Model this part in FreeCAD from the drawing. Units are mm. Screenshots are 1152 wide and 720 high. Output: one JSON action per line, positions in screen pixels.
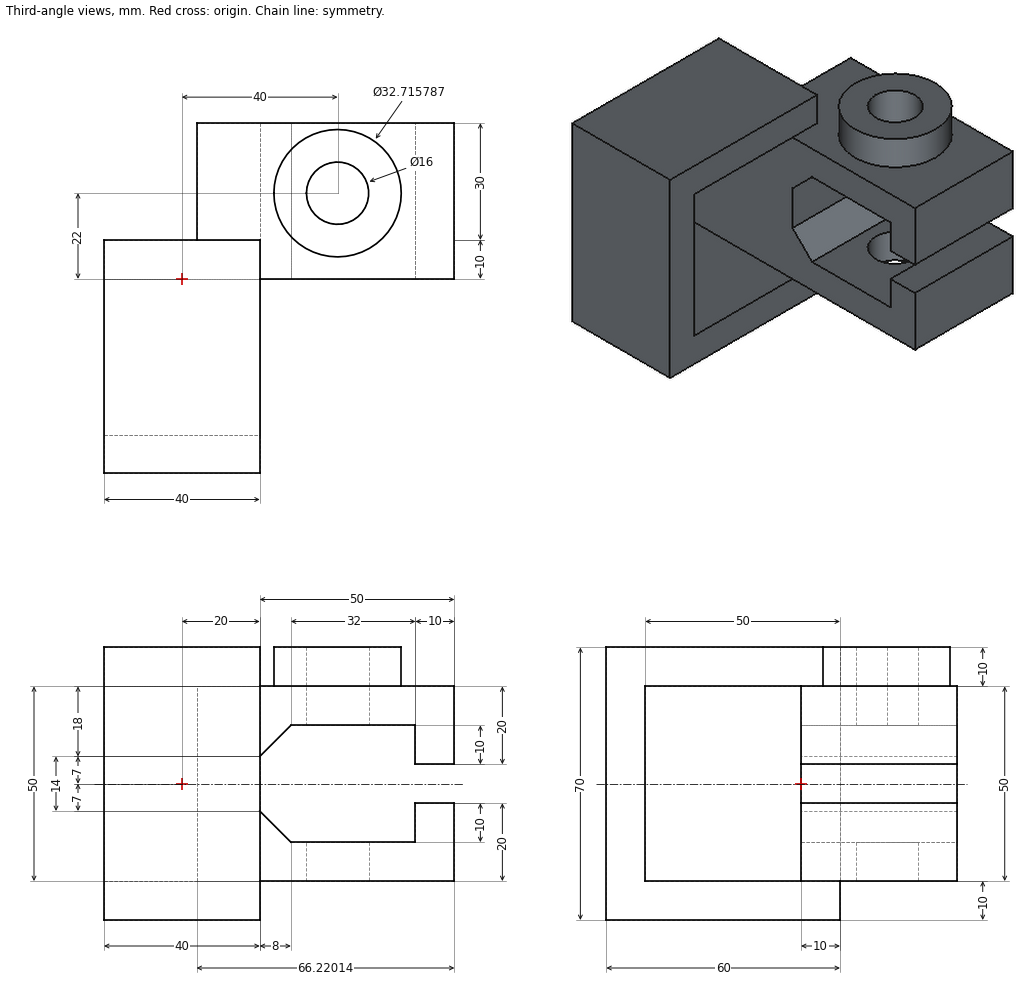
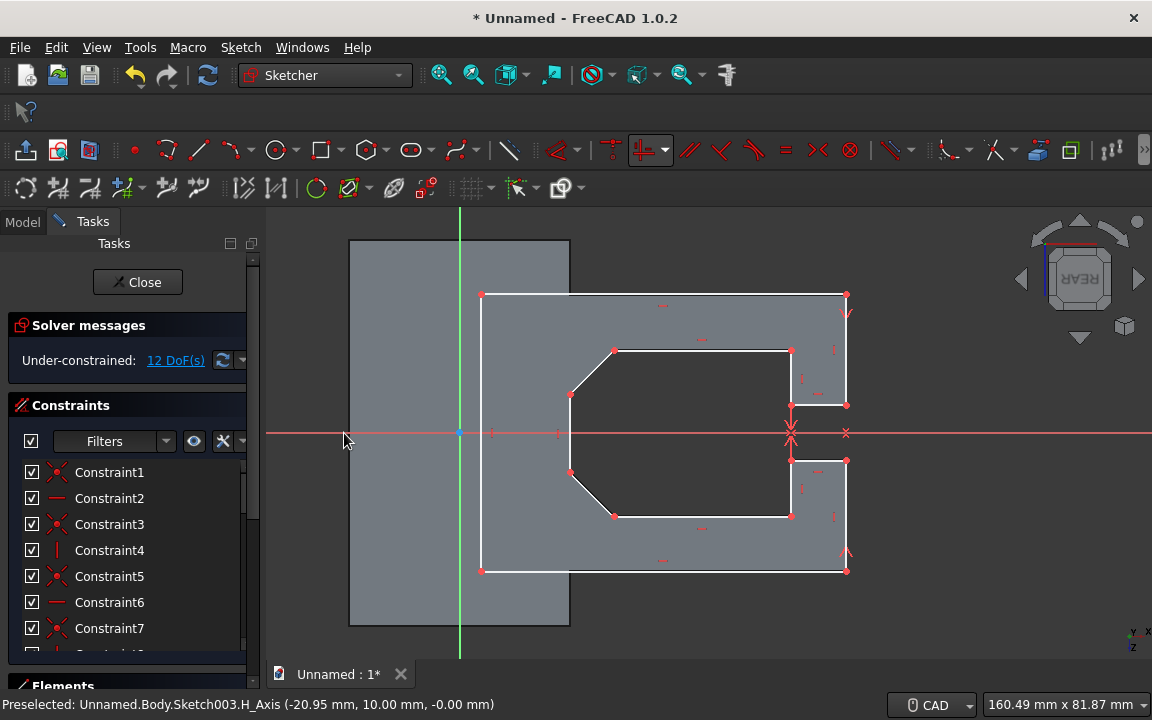
{"action": "left_click", "coordinate": [614, 351]}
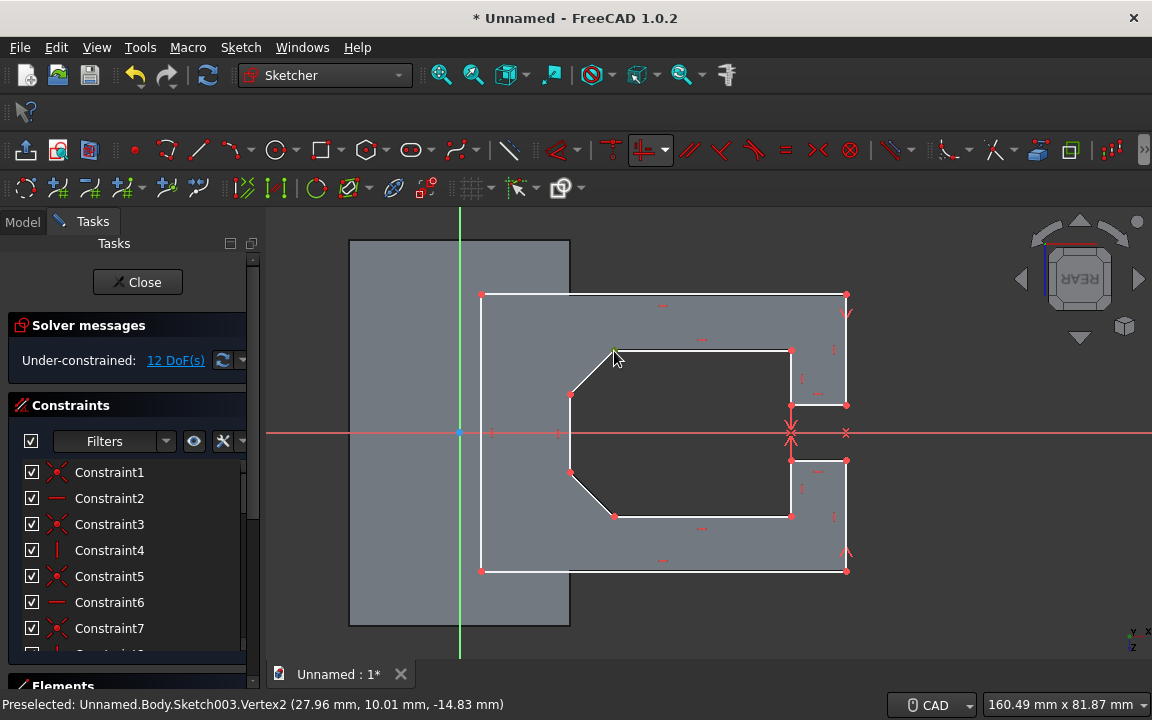
{"action": "left_click", "coordinate": [614, 517]}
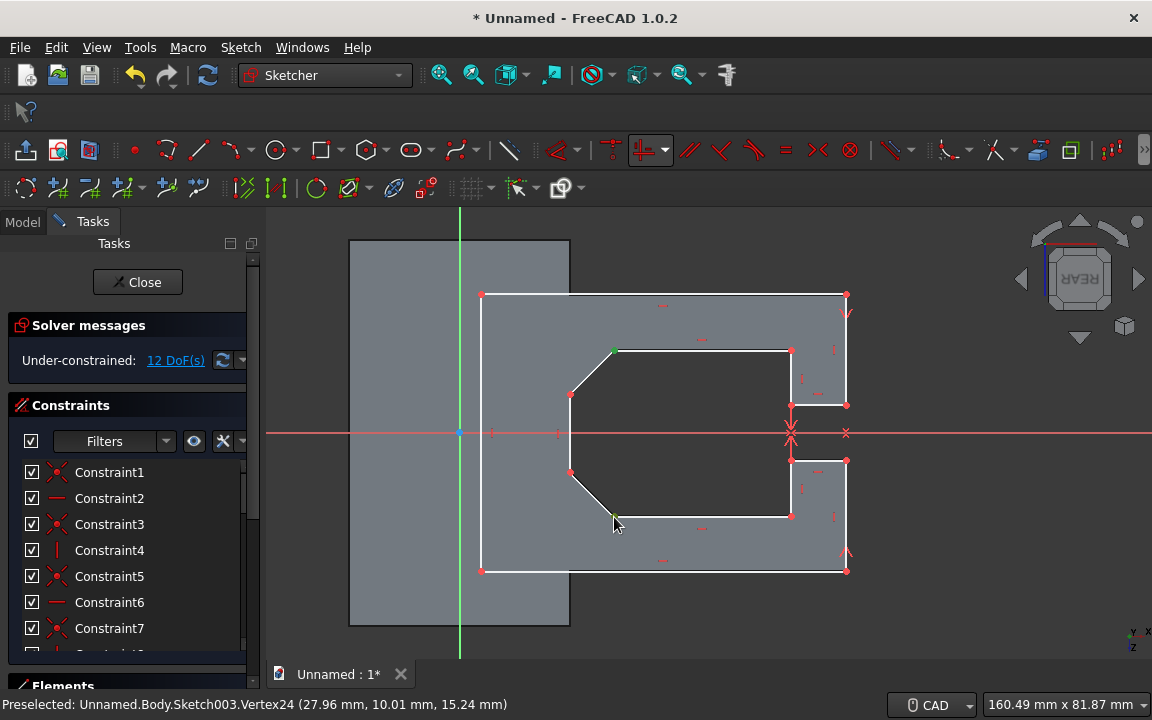
{"action": "left_click", "coordinate": [344, 433]}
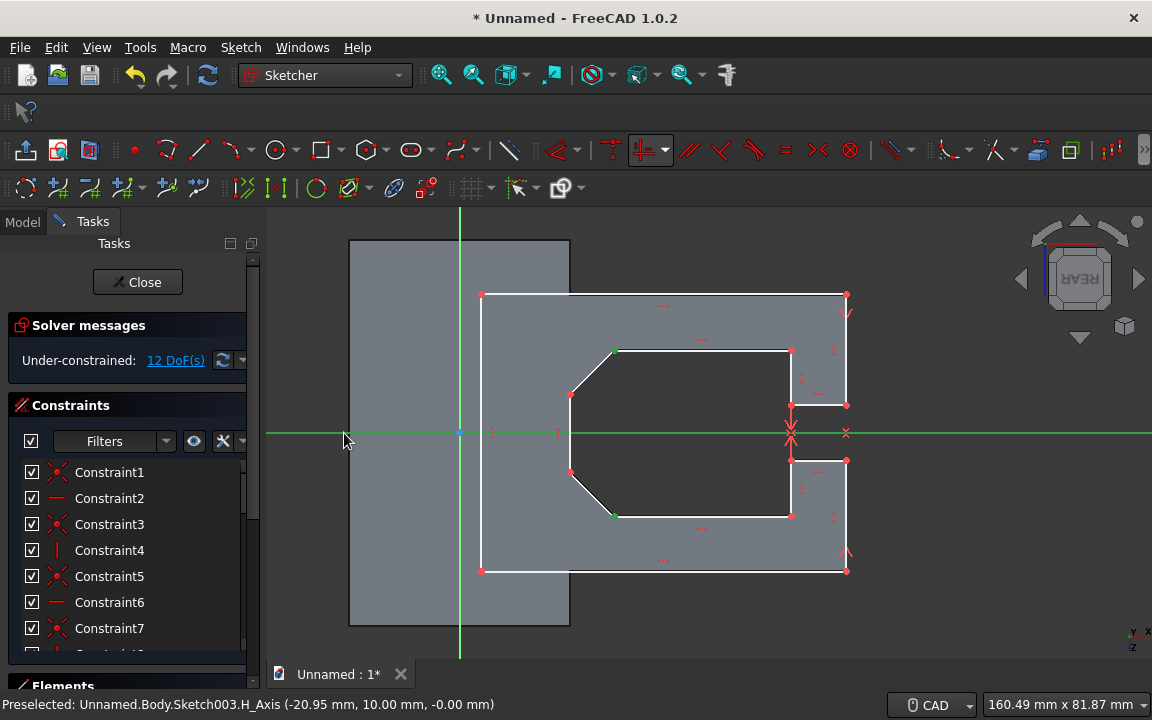
{"action": "key", "text": "s"}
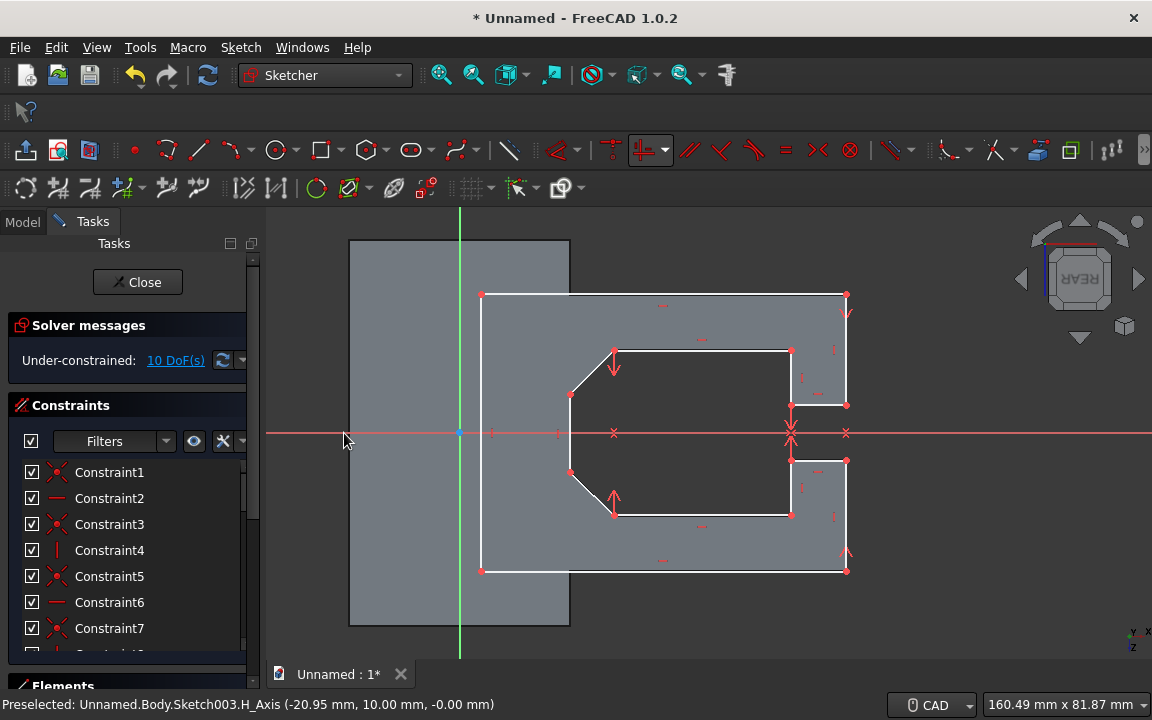
{"action": "key", "text": "d"}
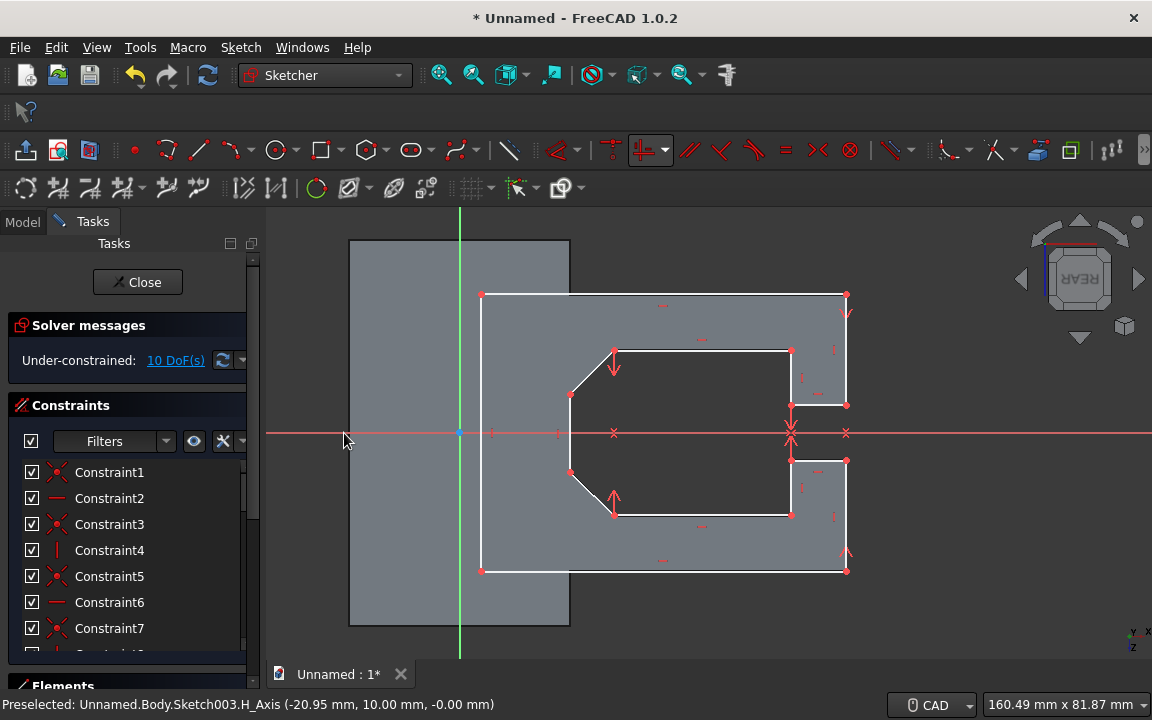
{"action": "left_click", "coordinate": [667, 351]}
{"action": "left_click", "coordinate": [703, 317]}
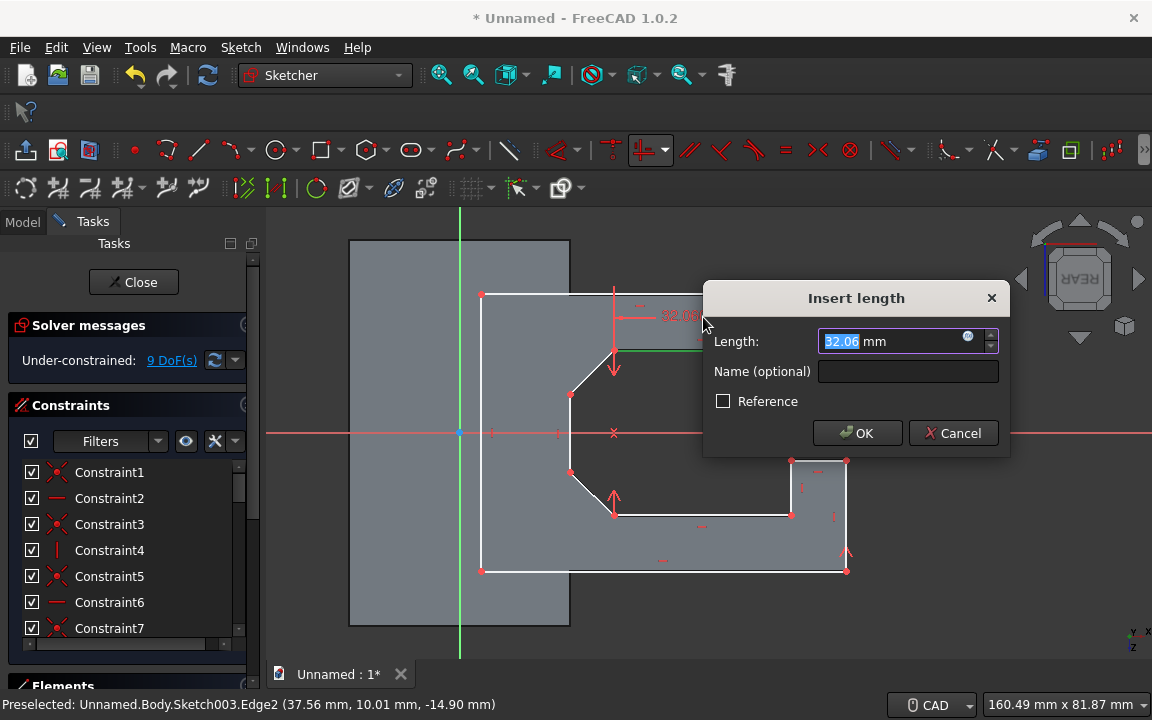
{"action": "type", "text": "32"}
{"action": "key", "text": "Return"}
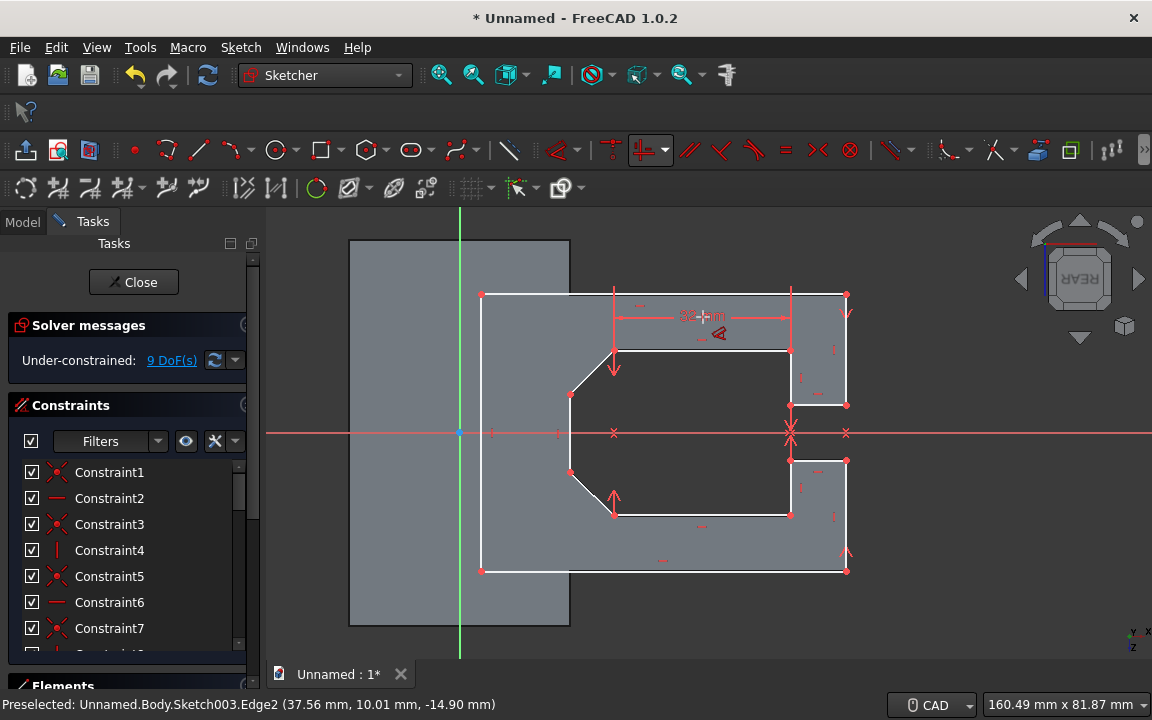
{"action": "left_click", "coordinate": [791, 367]}
{"action": "left_click", "coordinate": [825, 378]}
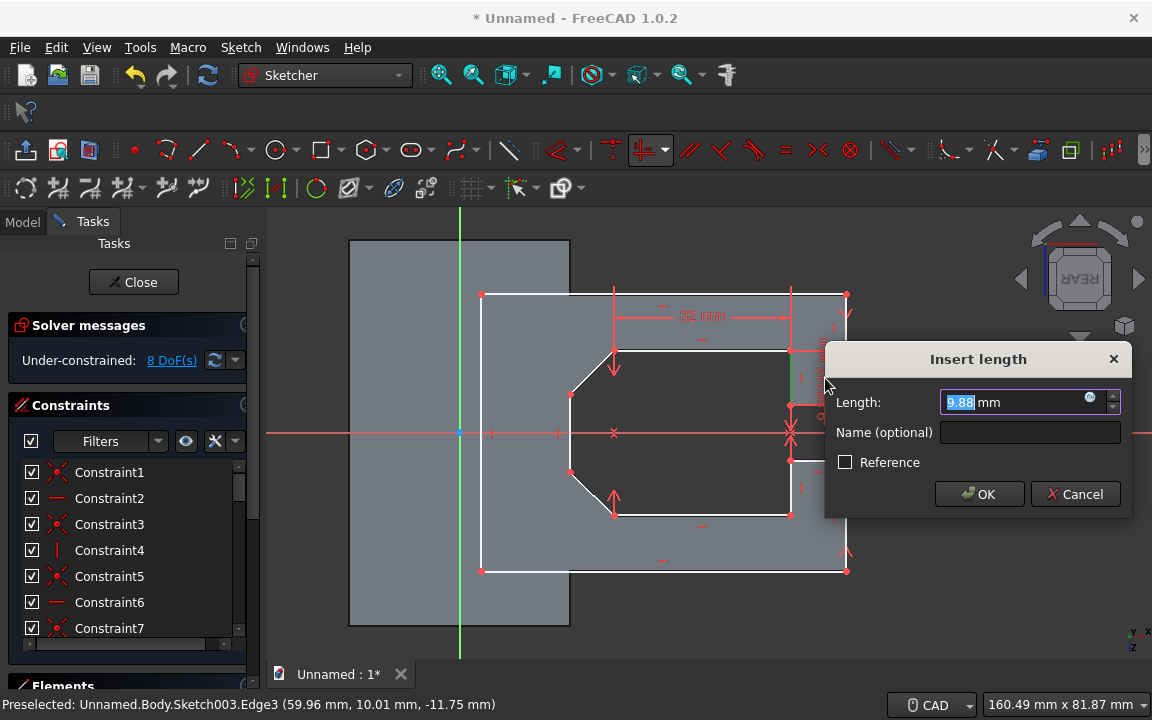
{"action": "type", "text": "10"}
{"action": "key", "text": "Return"}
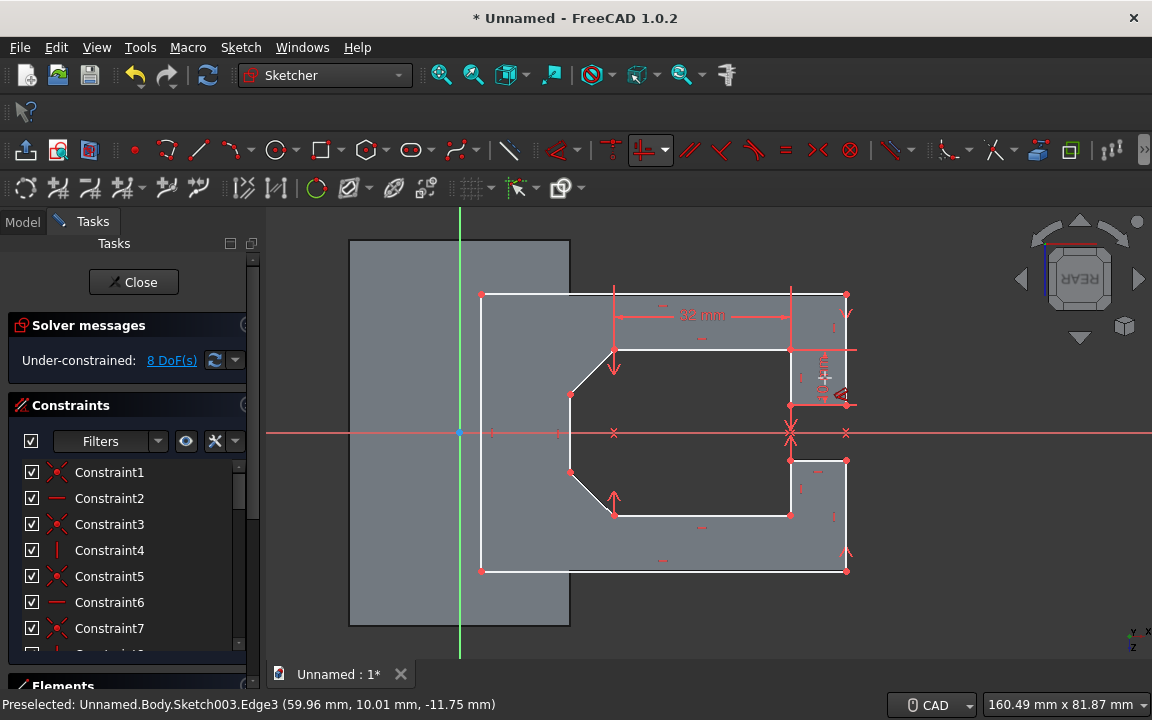
{"action": "left_click", "coordinate": [807, 405]}
{"action": "left_click", "coordinate": [818, 347]}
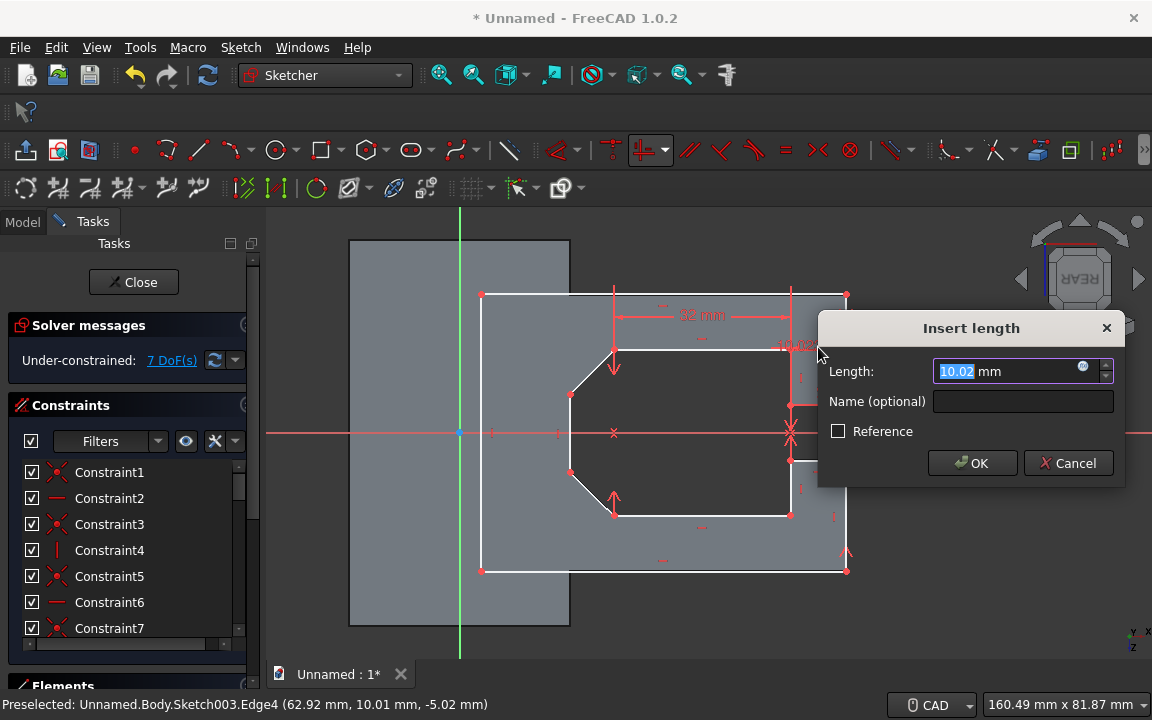
{"action": "type", "text": "10"}
{"action": "key", "text": "Return"}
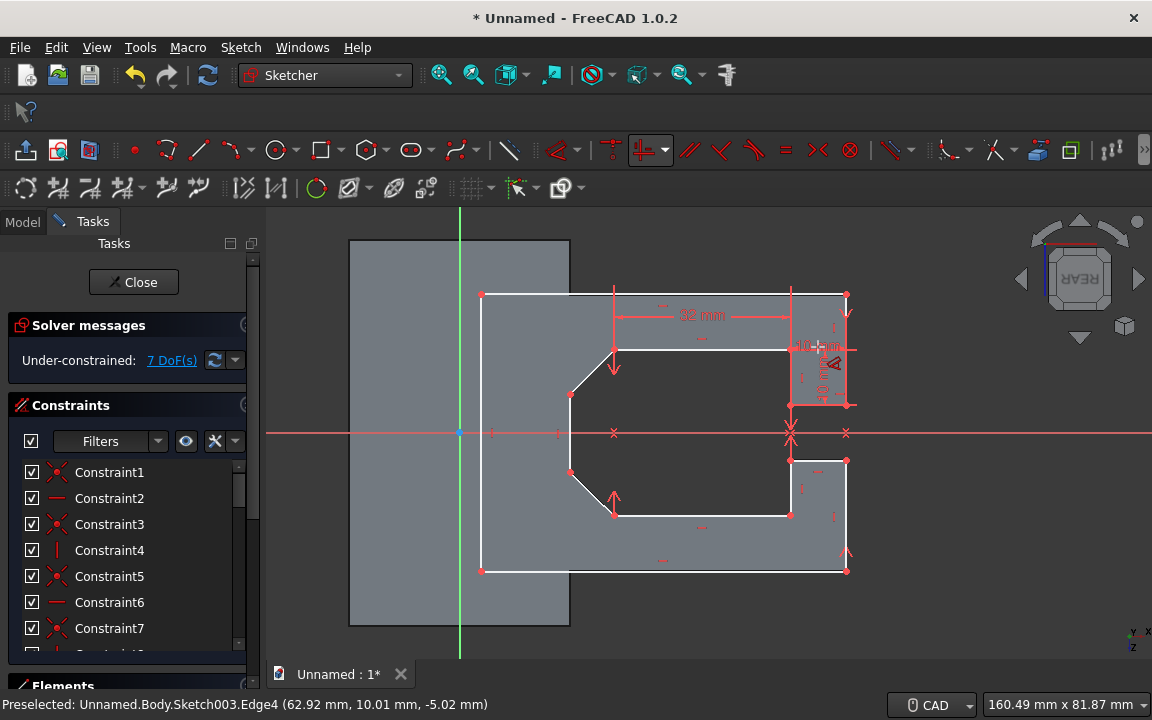
{"action": "left_click", "coordinate": [846, 372]}
{"action": "left_click", "coordinate": [880, 324]}